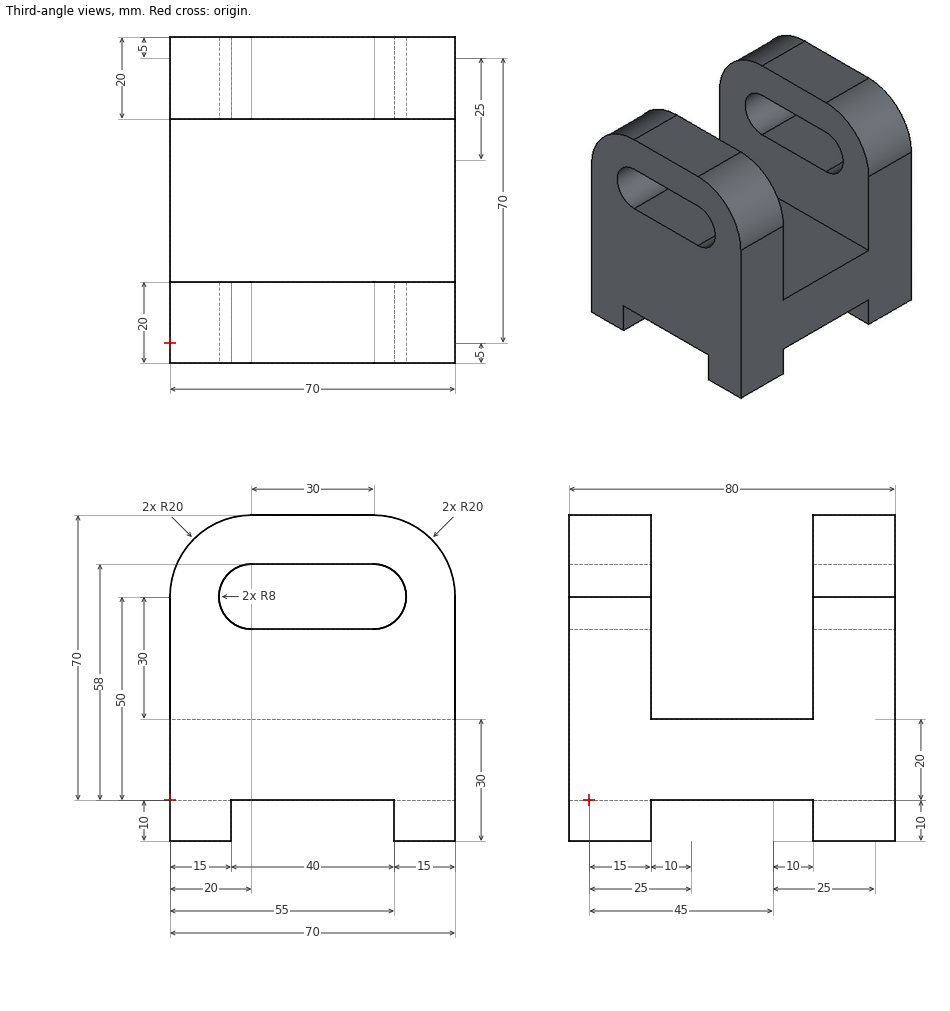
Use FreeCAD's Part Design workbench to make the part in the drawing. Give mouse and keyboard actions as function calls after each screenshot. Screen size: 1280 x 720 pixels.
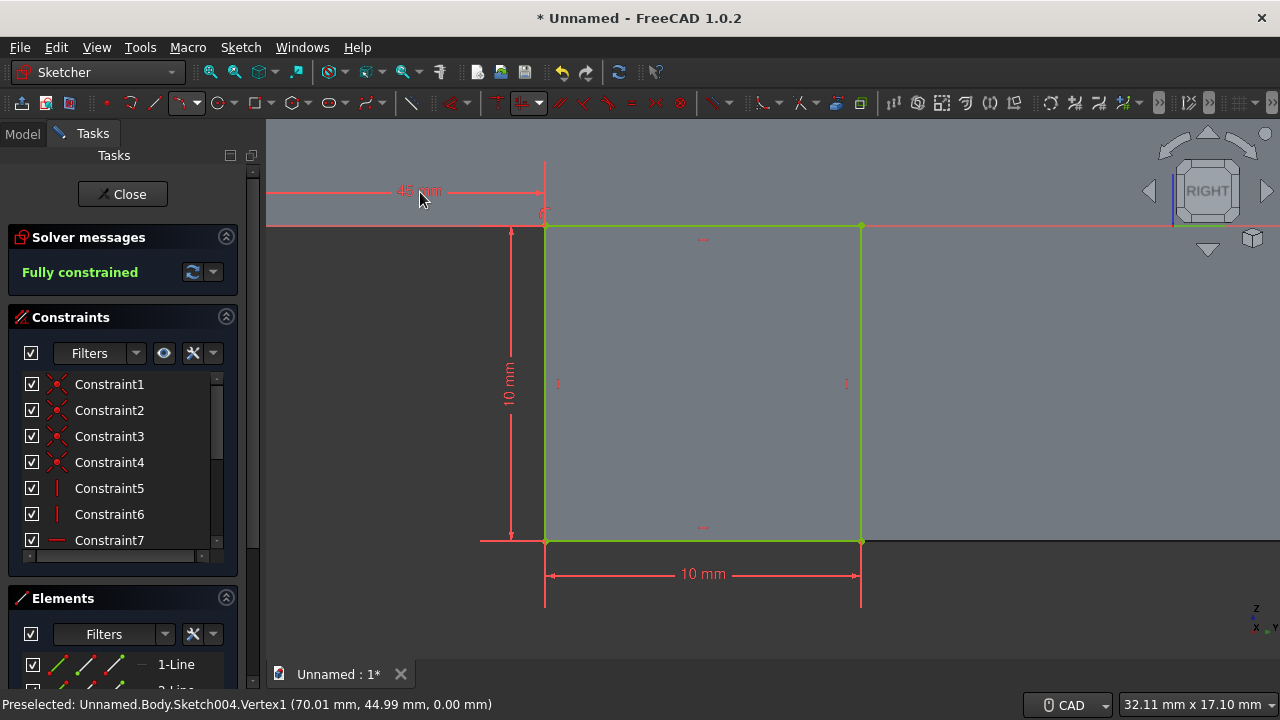
click(123, 194)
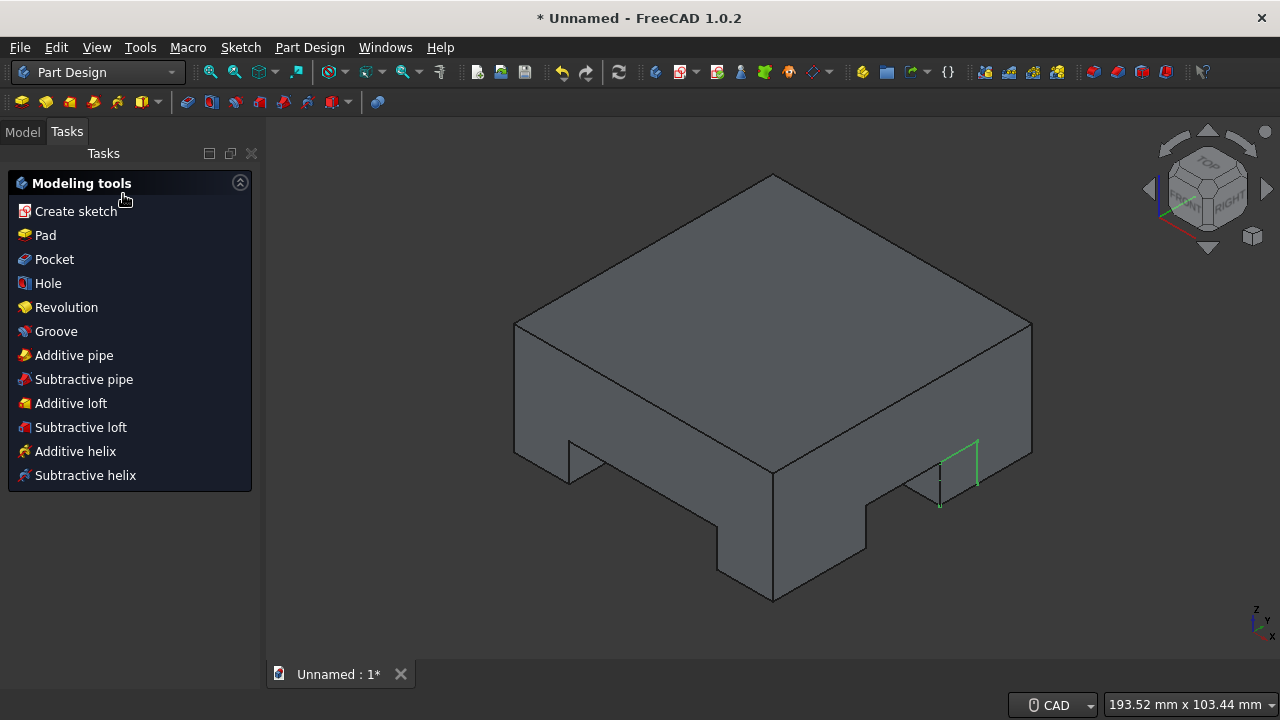
click(188, 102)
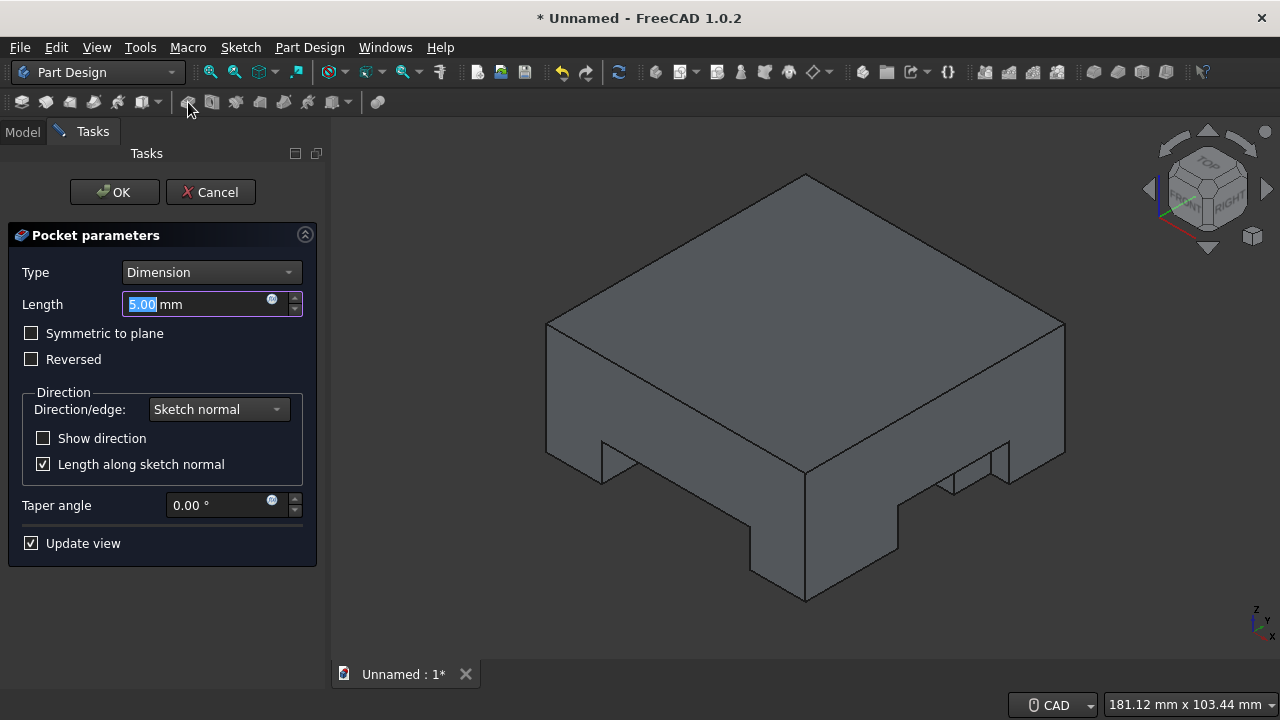
text(70)
key(Tab)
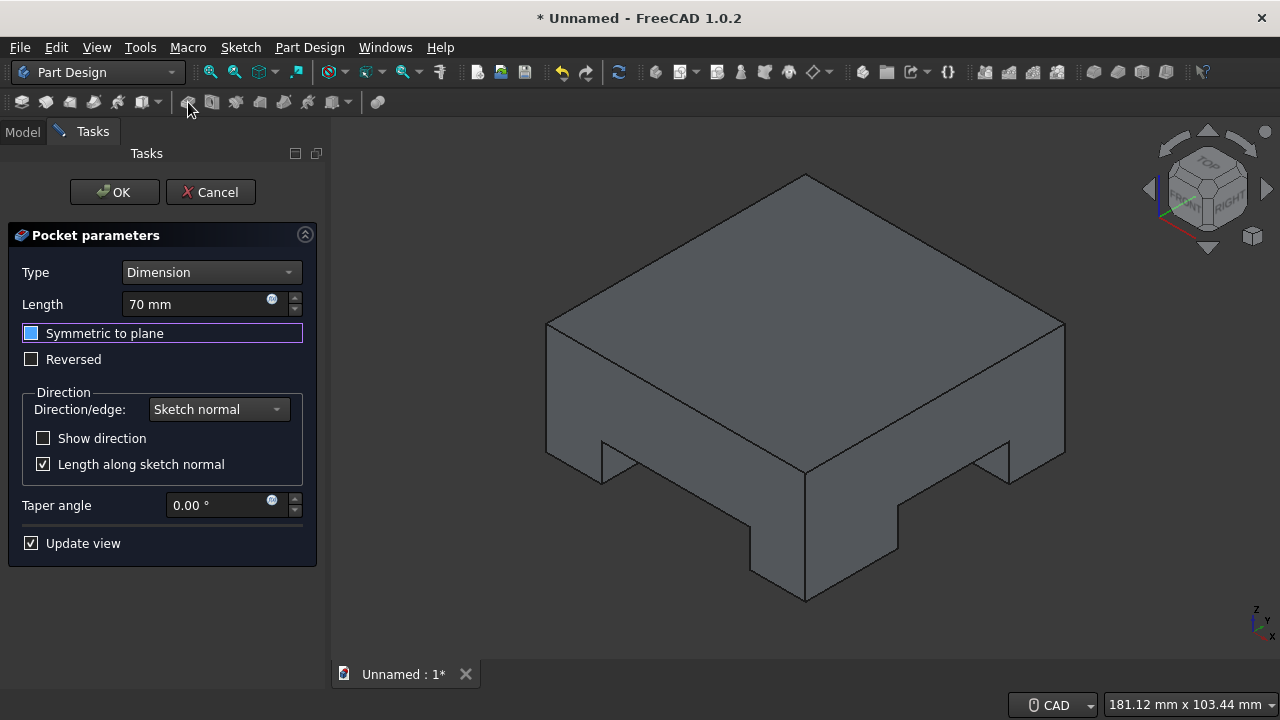
click(115, 192)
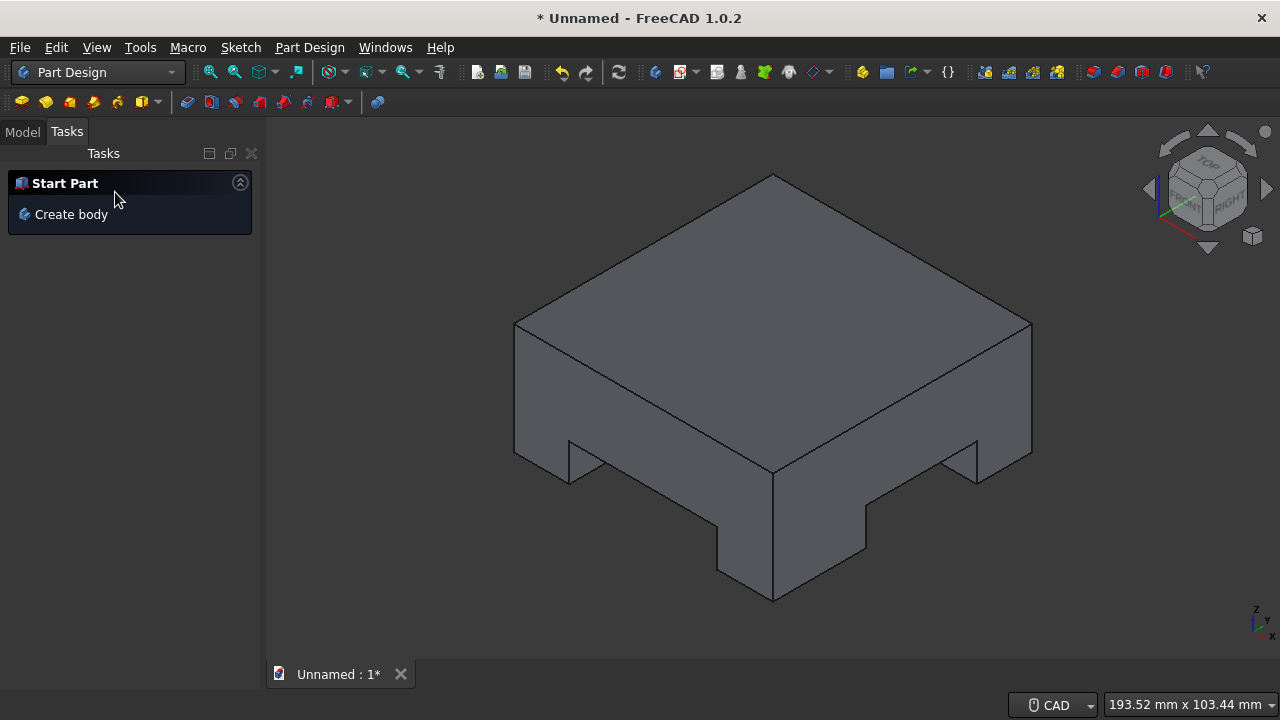
click(829, 505)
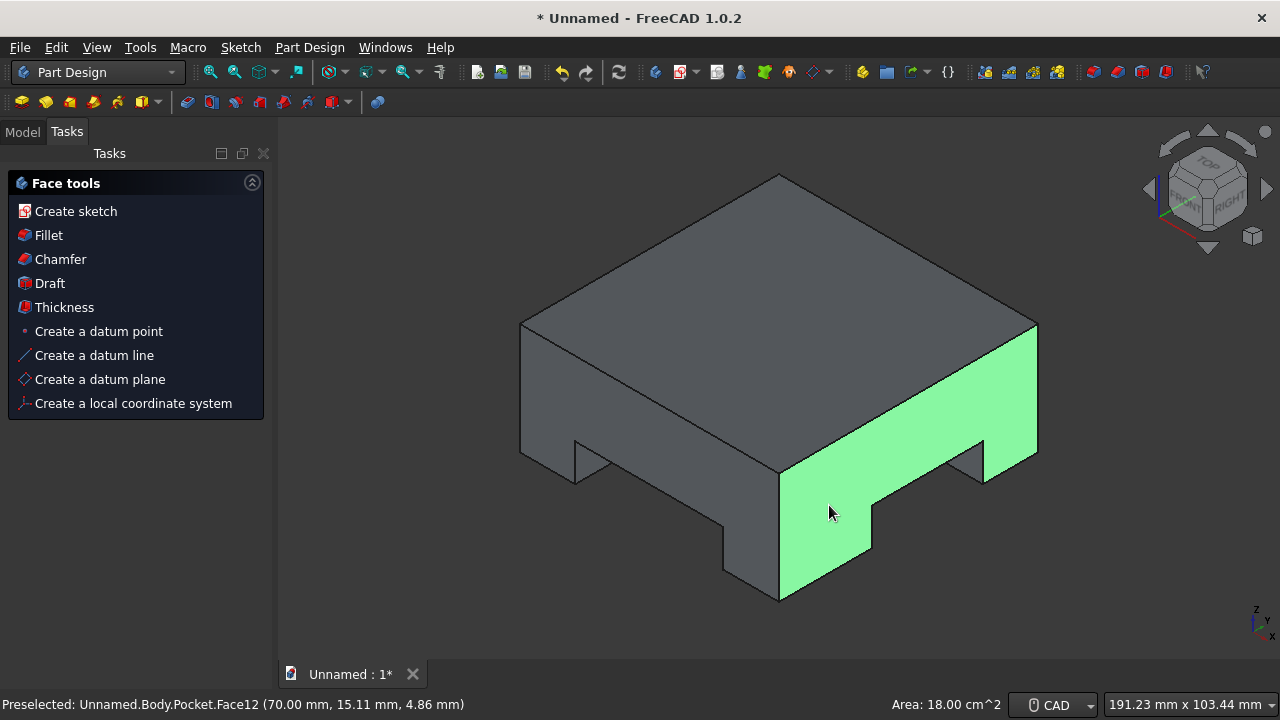
click(680, 72)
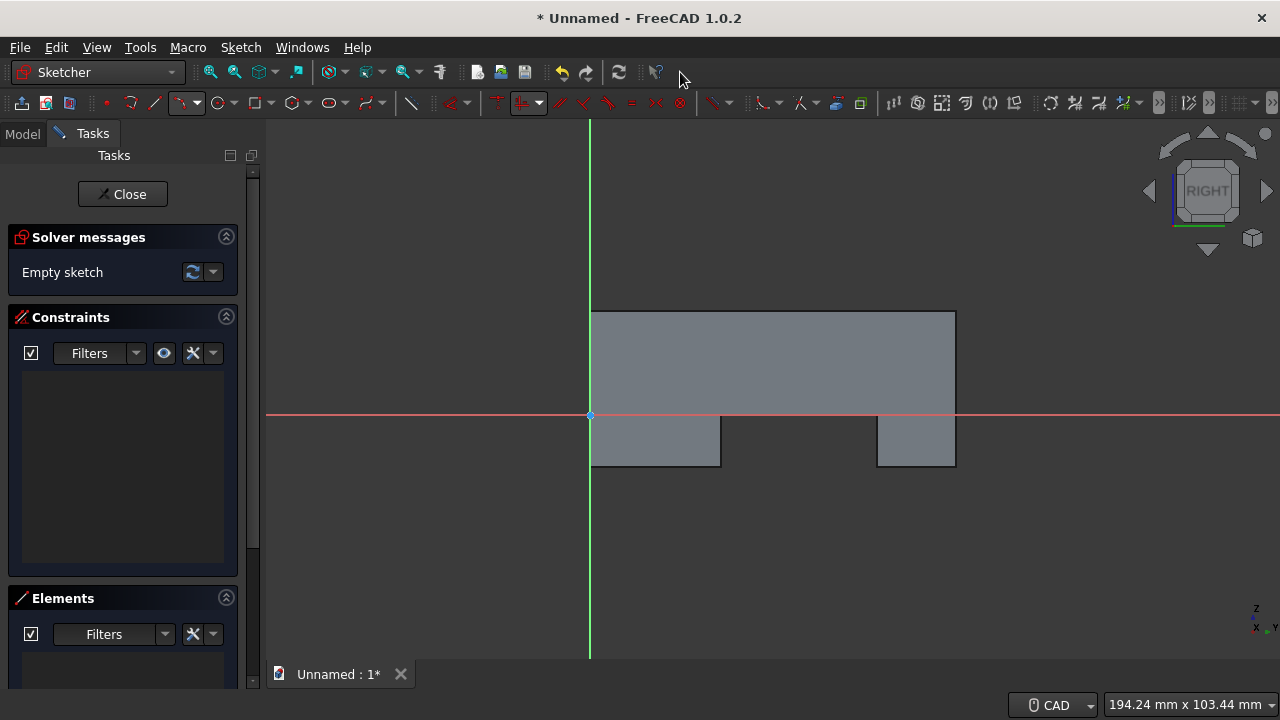
scroll(693, 452, up, 9)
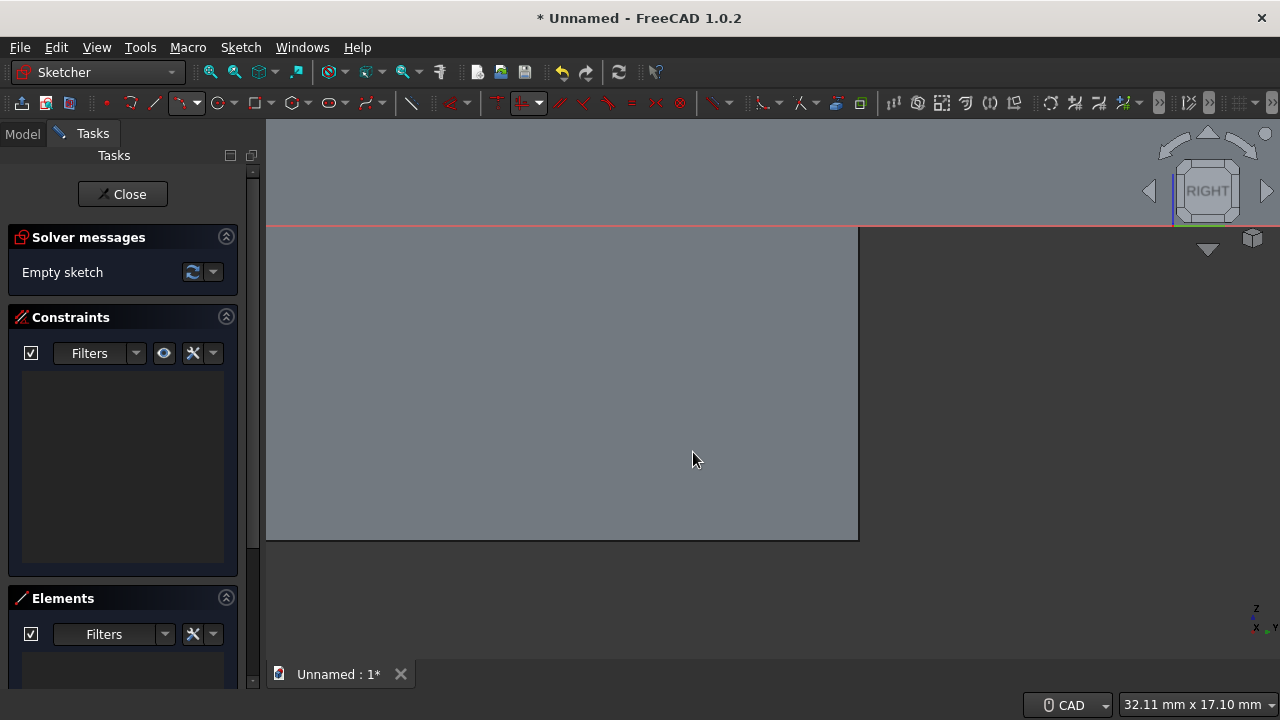
key(g)
key(r)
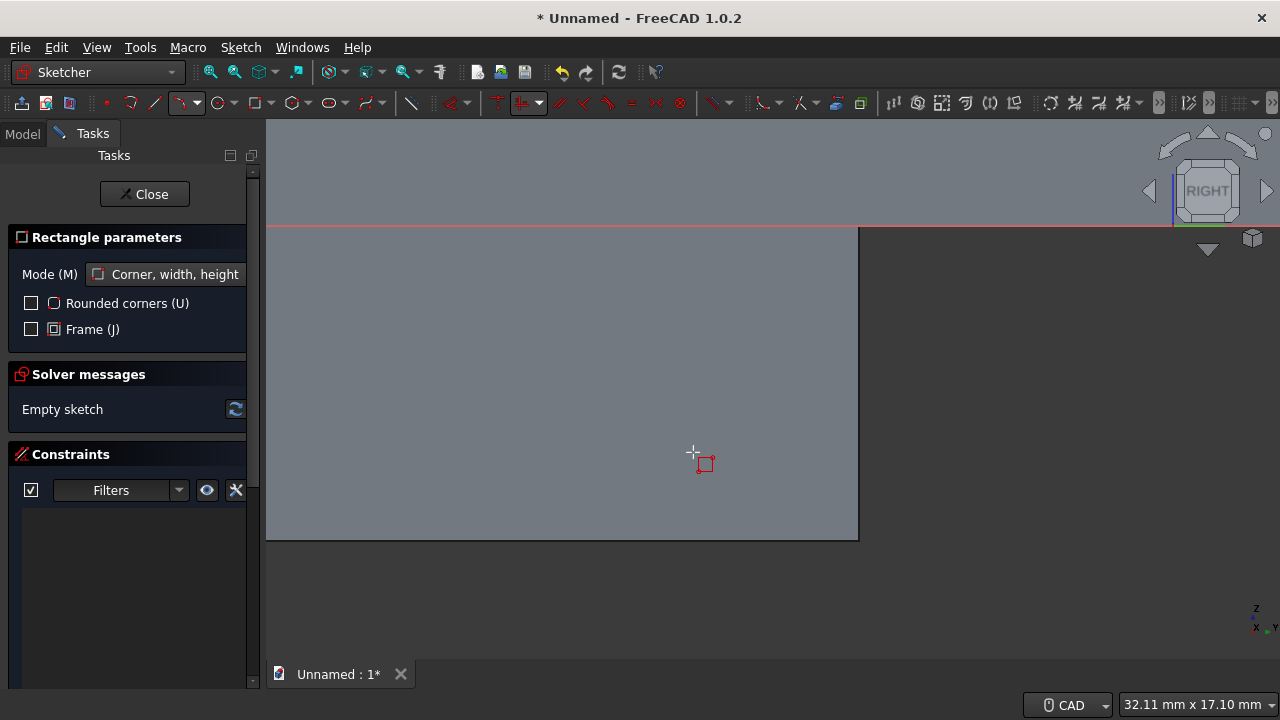
click(543, 226)
click(859, 541)
key(Escape)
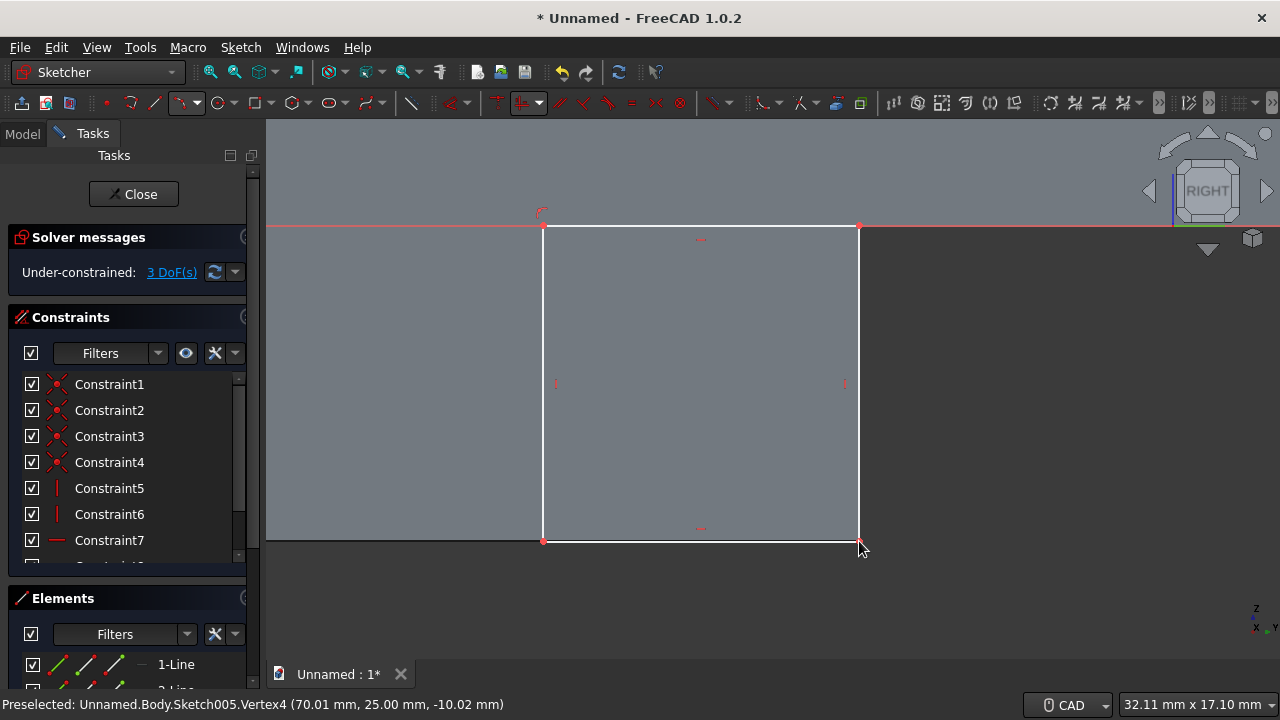
key(d)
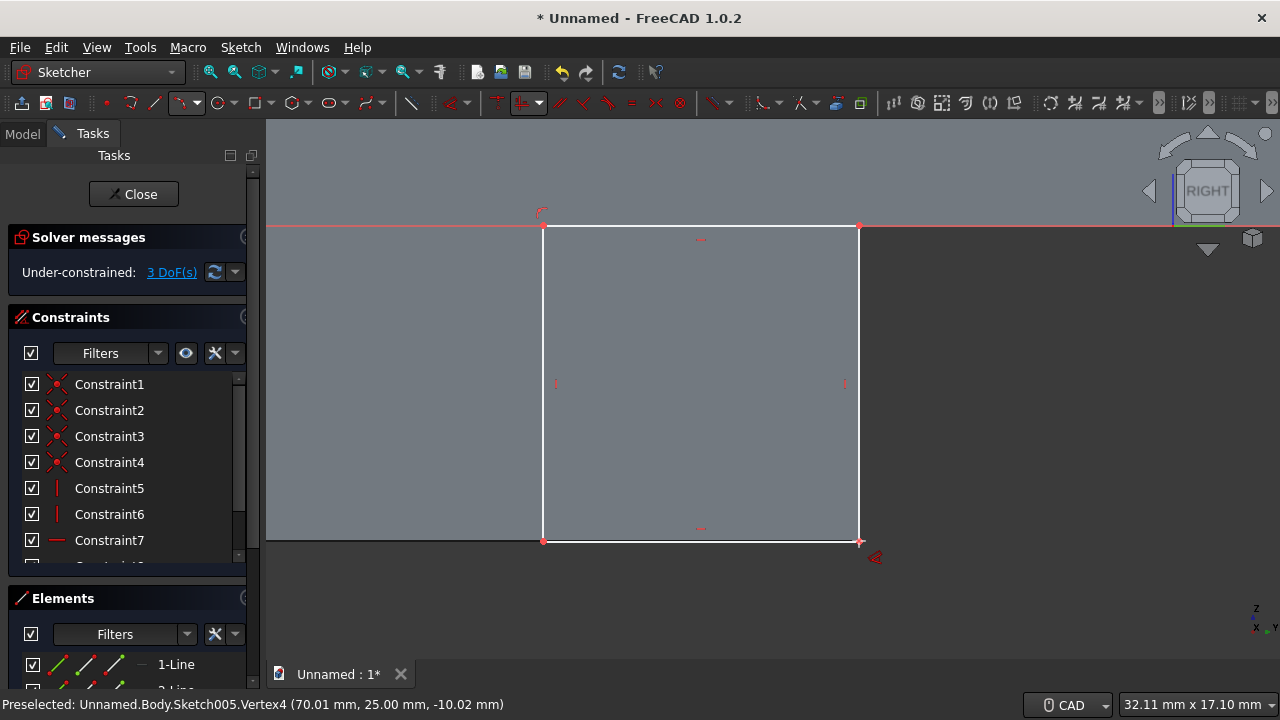
click(543, 321)
click(509, 384)